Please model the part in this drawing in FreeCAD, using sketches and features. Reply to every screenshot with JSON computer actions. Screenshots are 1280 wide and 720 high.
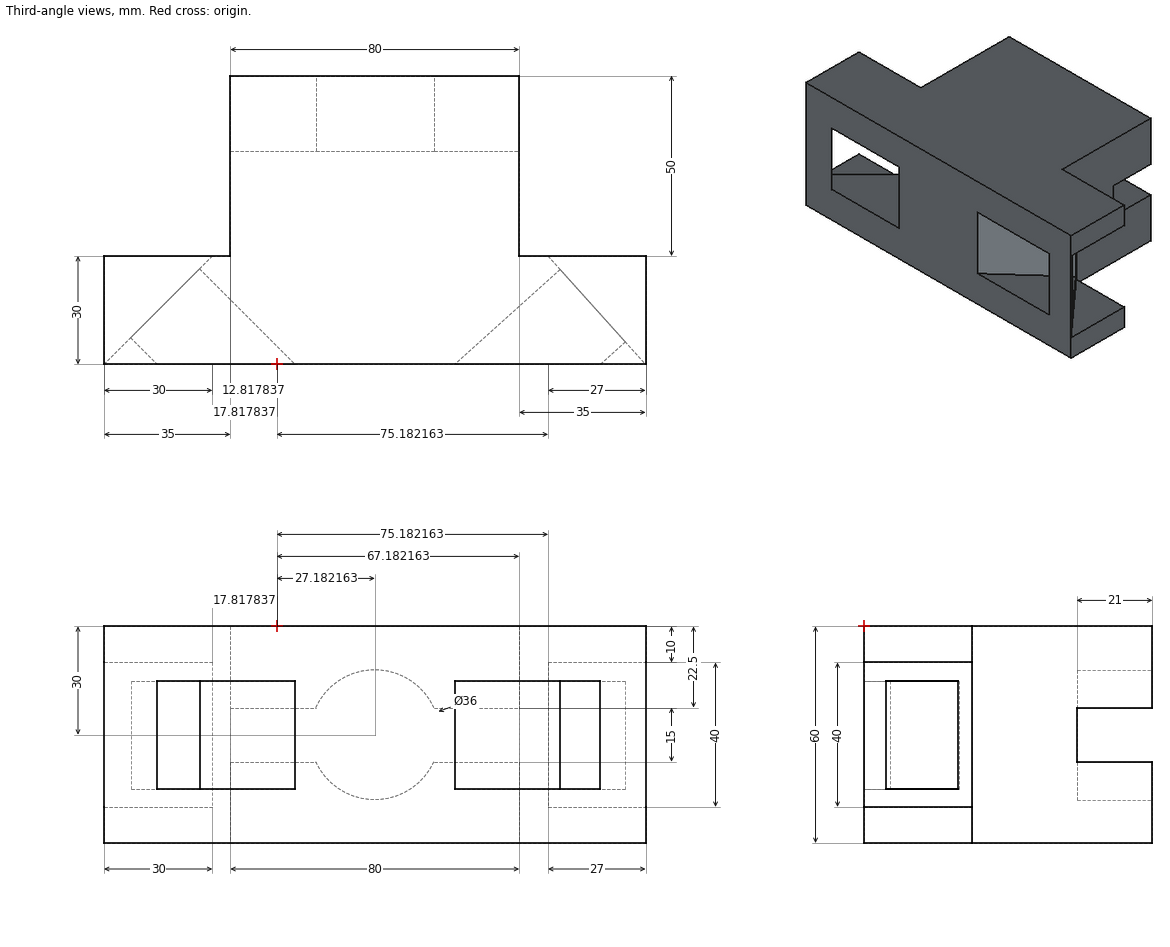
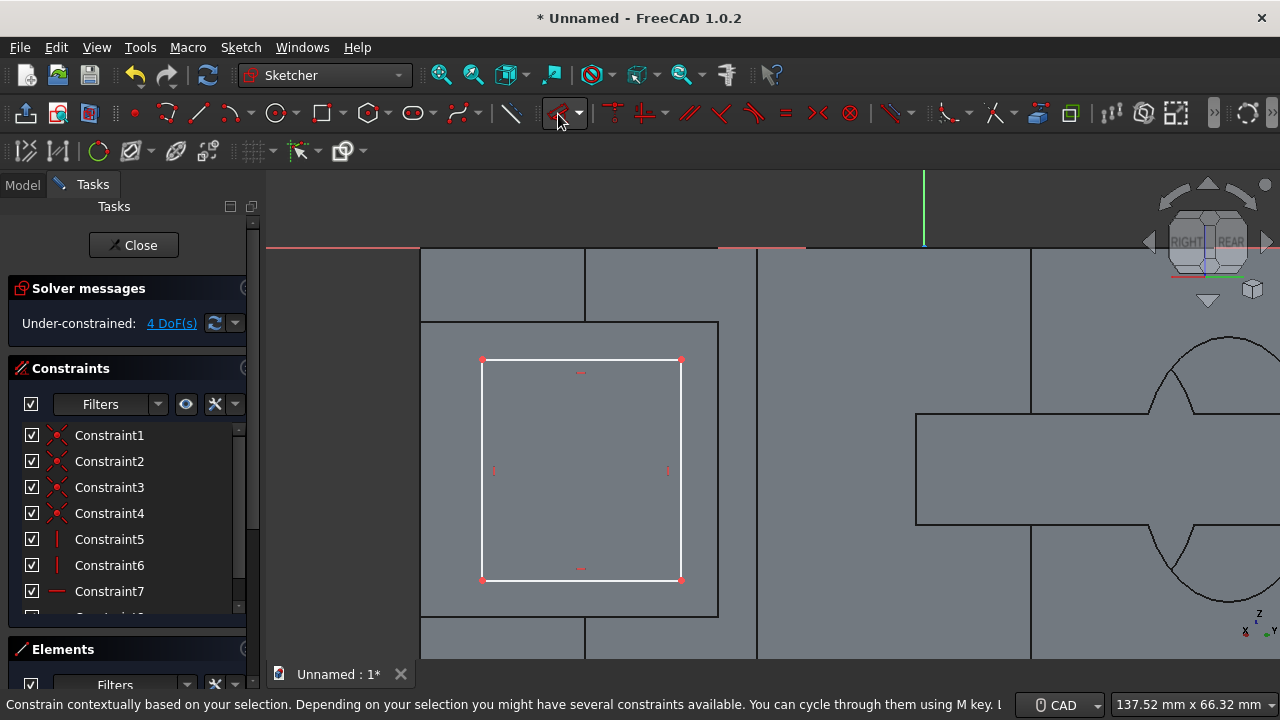
{"action": "left_click", "coordinate": [482, 426]}
{"action": "left_click", "coordinate": [448, 471]}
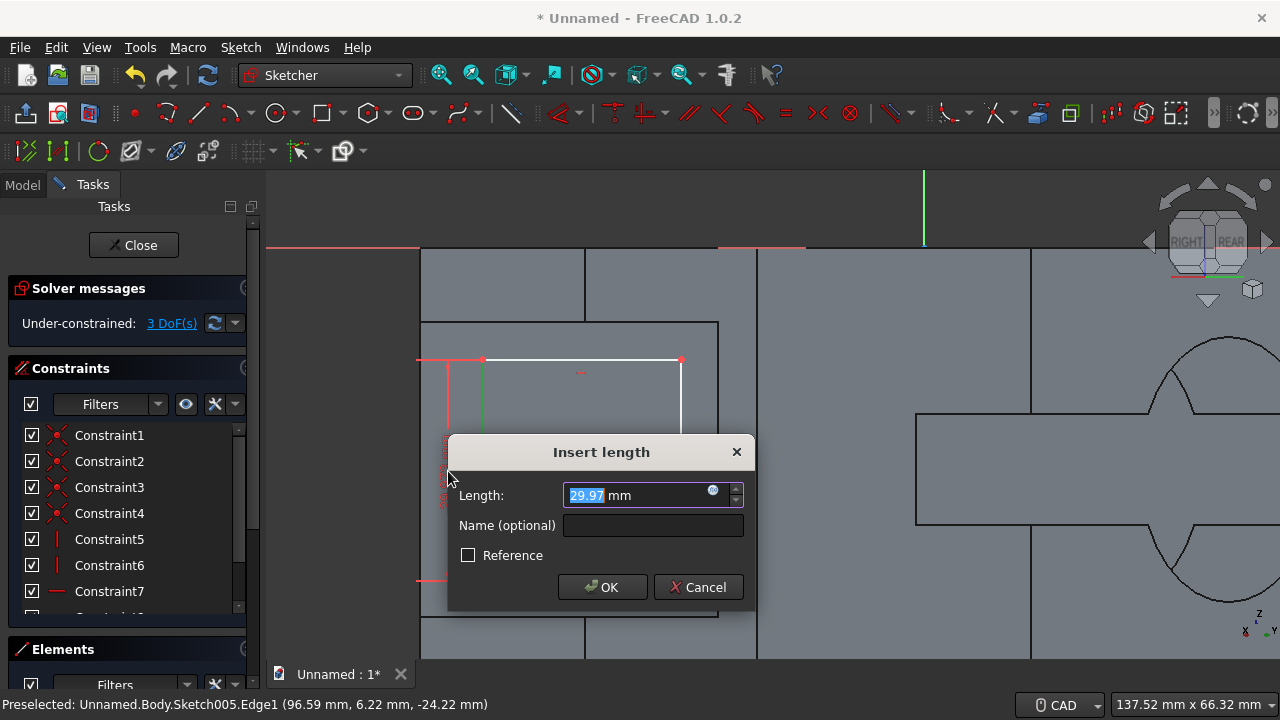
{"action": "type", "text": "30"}
{"action": "key", "text": "Return"}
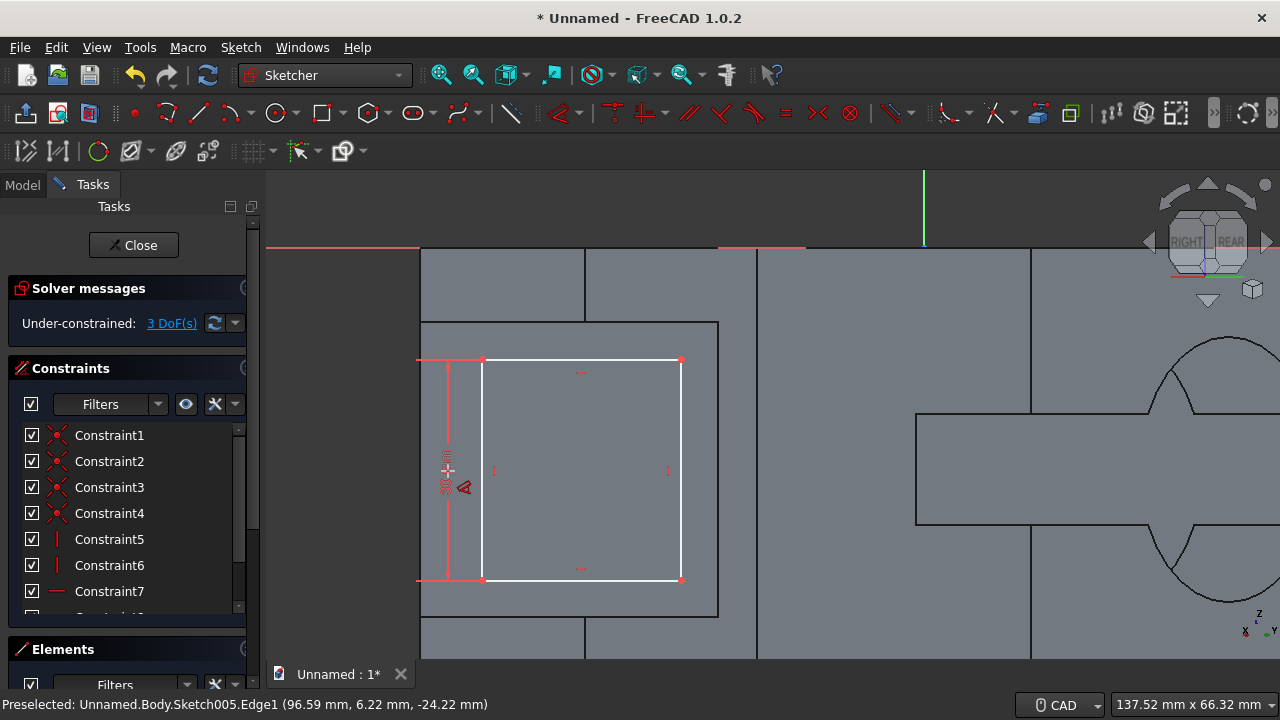
{"action": "left_click", "coordinate": [542, 581]}
{"action": "left_click", "coordinate": [581, 615]}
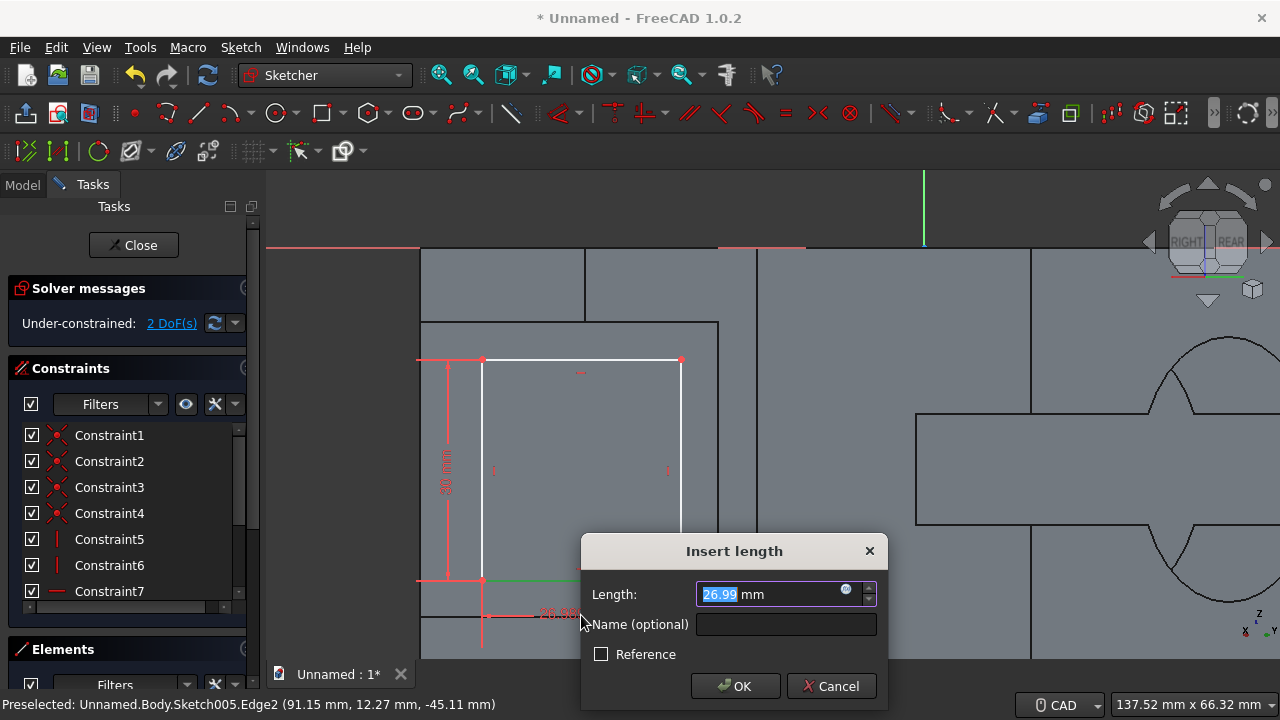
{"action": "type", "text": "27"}
{"action": "key", "text": "Return"}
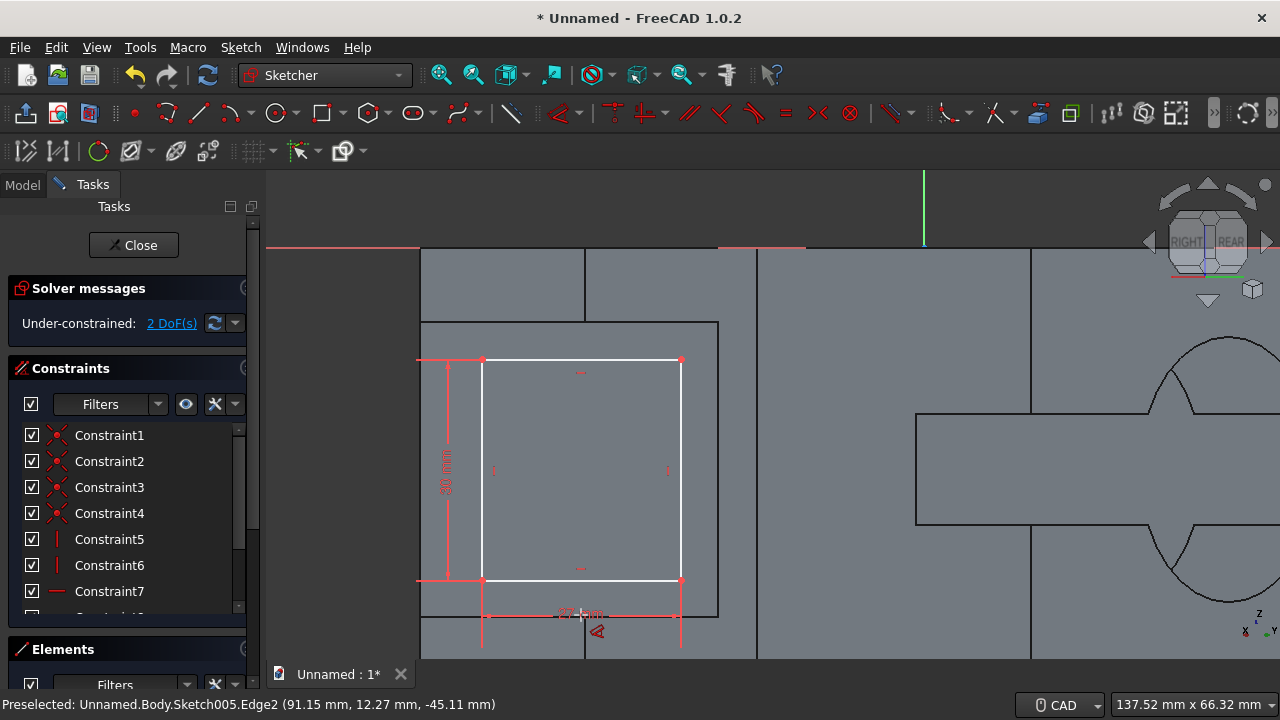
{"action": "left_click", "coordinate": [482, 360]}
{"action": "left_click", "coordinate": [958, 304]}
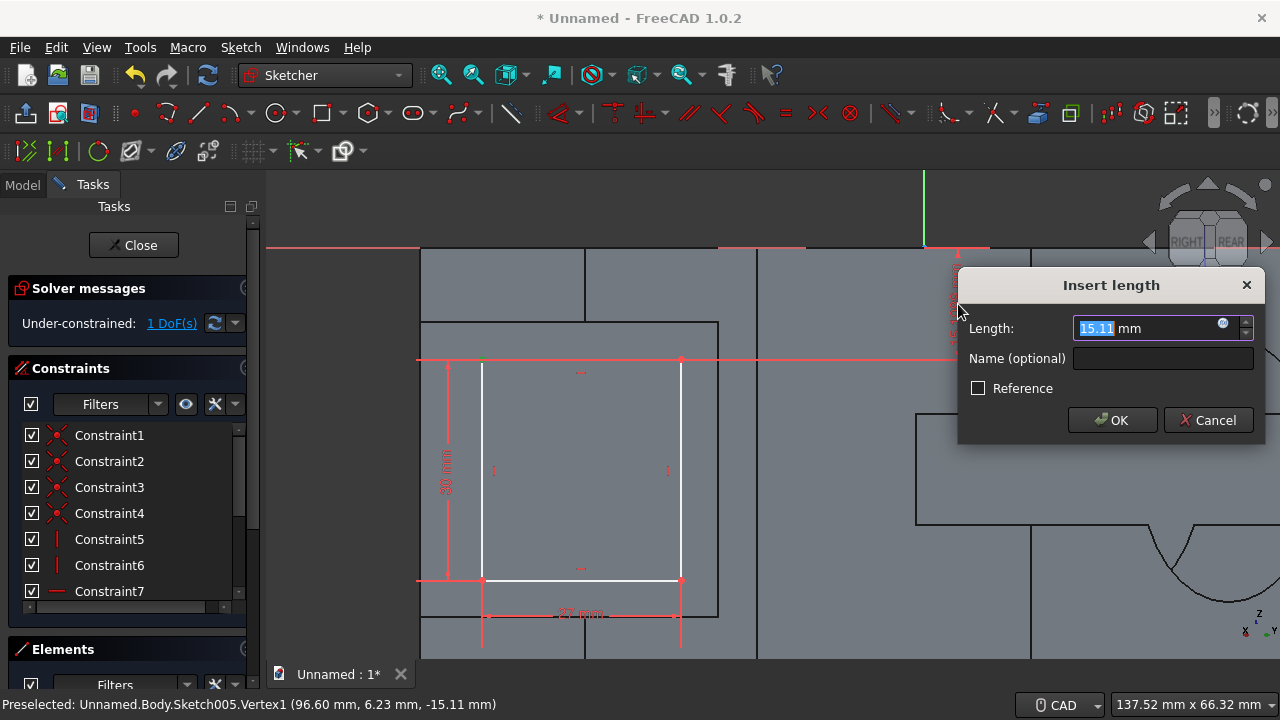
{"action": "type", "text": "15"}
{"action": "key", "text": "Return"}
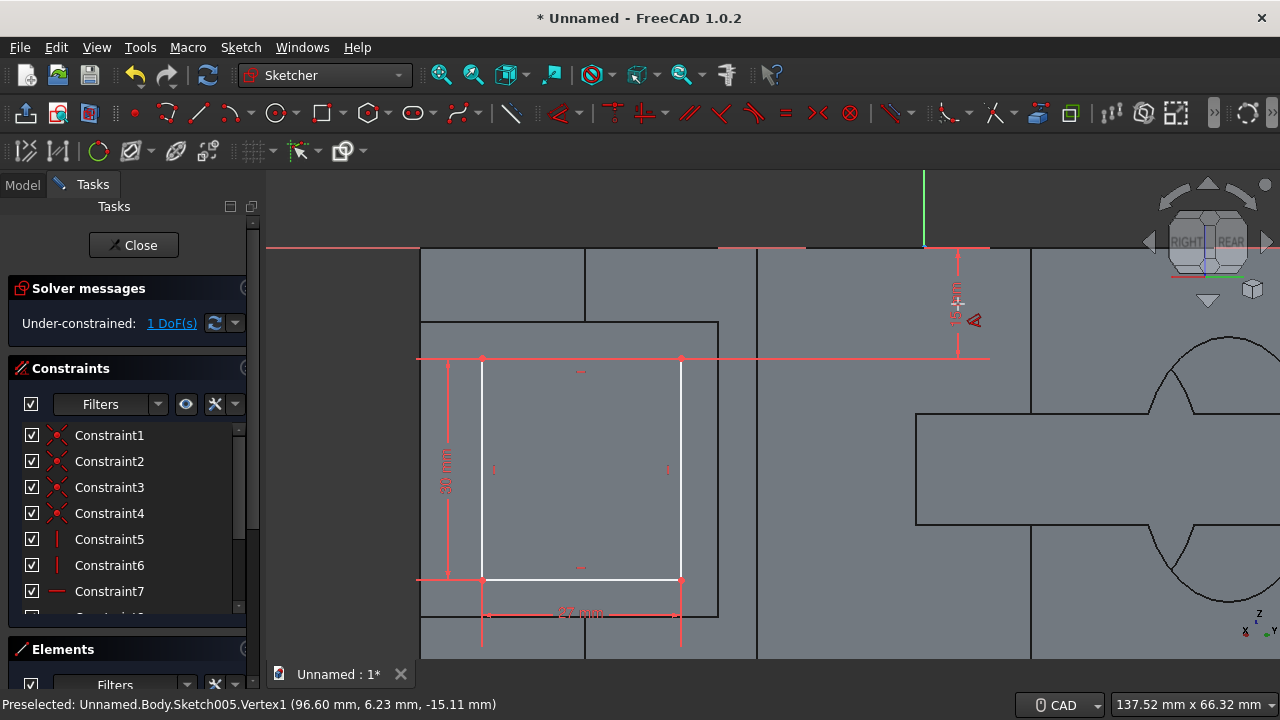
{"action": "left_click", "coordinate": [482, 359]}
{"action": "left_click", "coordinate": [703, 214]}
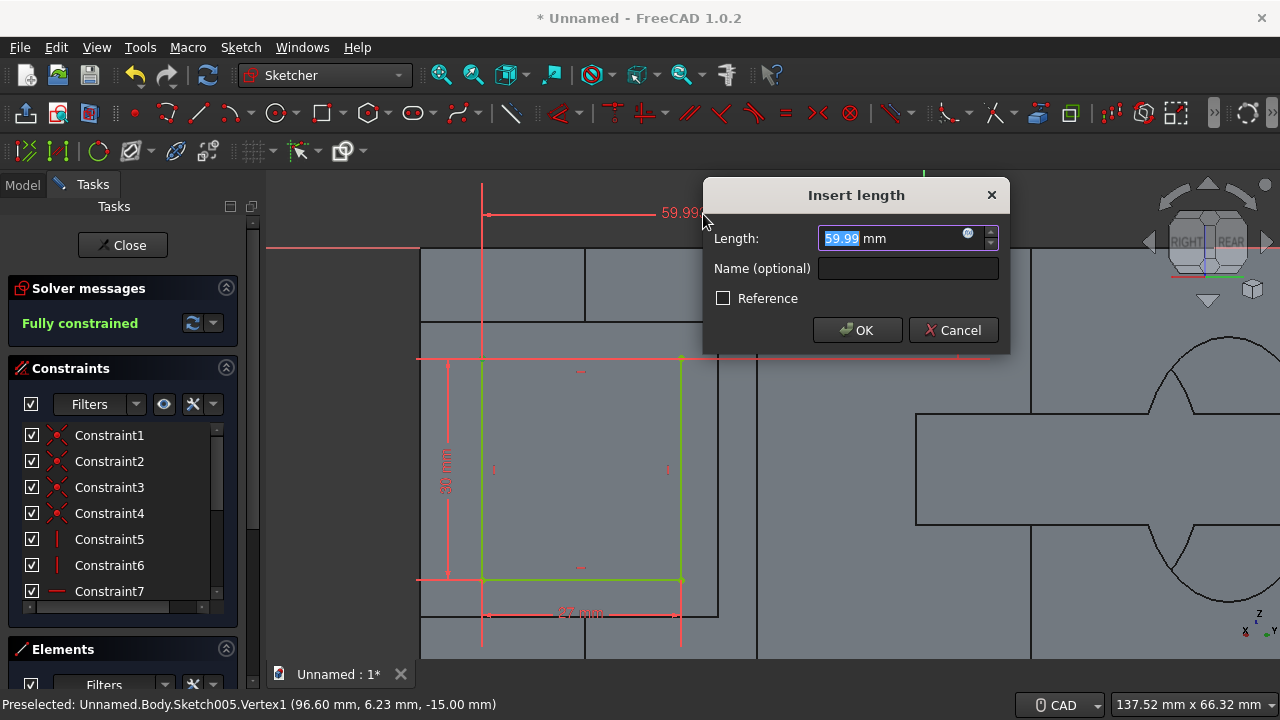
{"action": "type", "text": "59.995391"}
{"action": "key", "text": "Return"}
{"action": "key", "text": "Escape"}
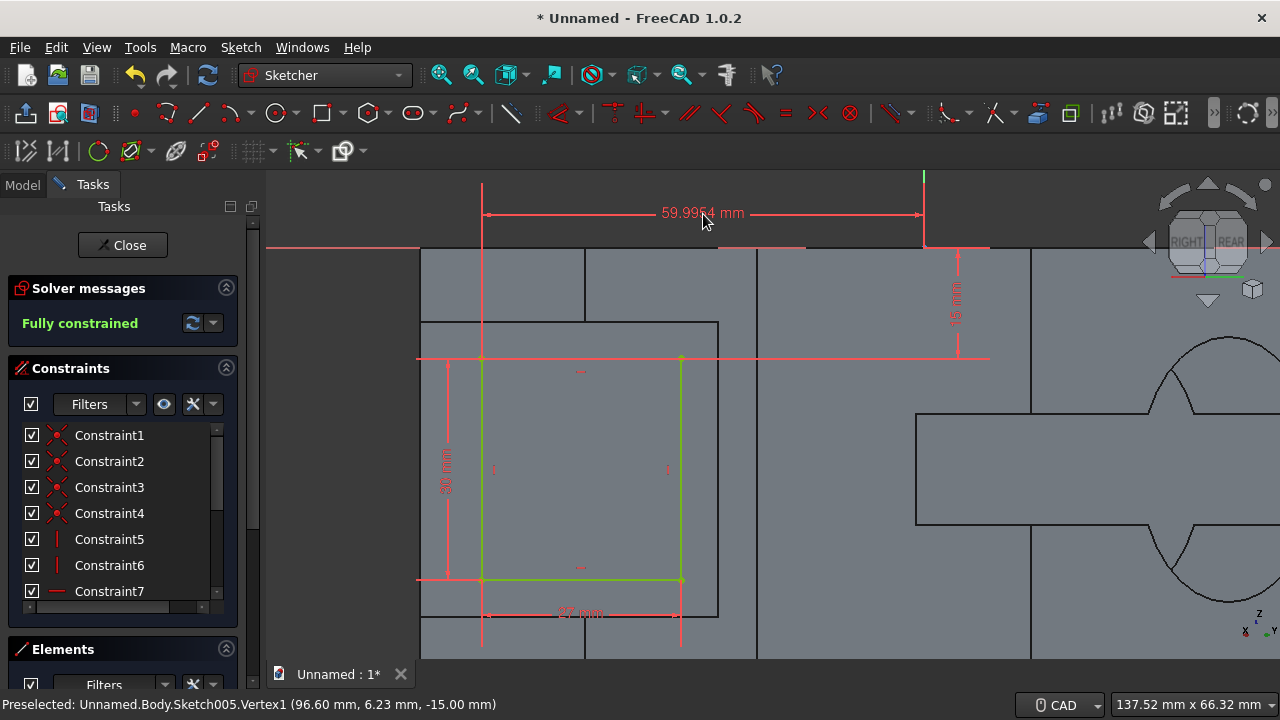
{"action": "left_click", "coordinate": [123, 245]}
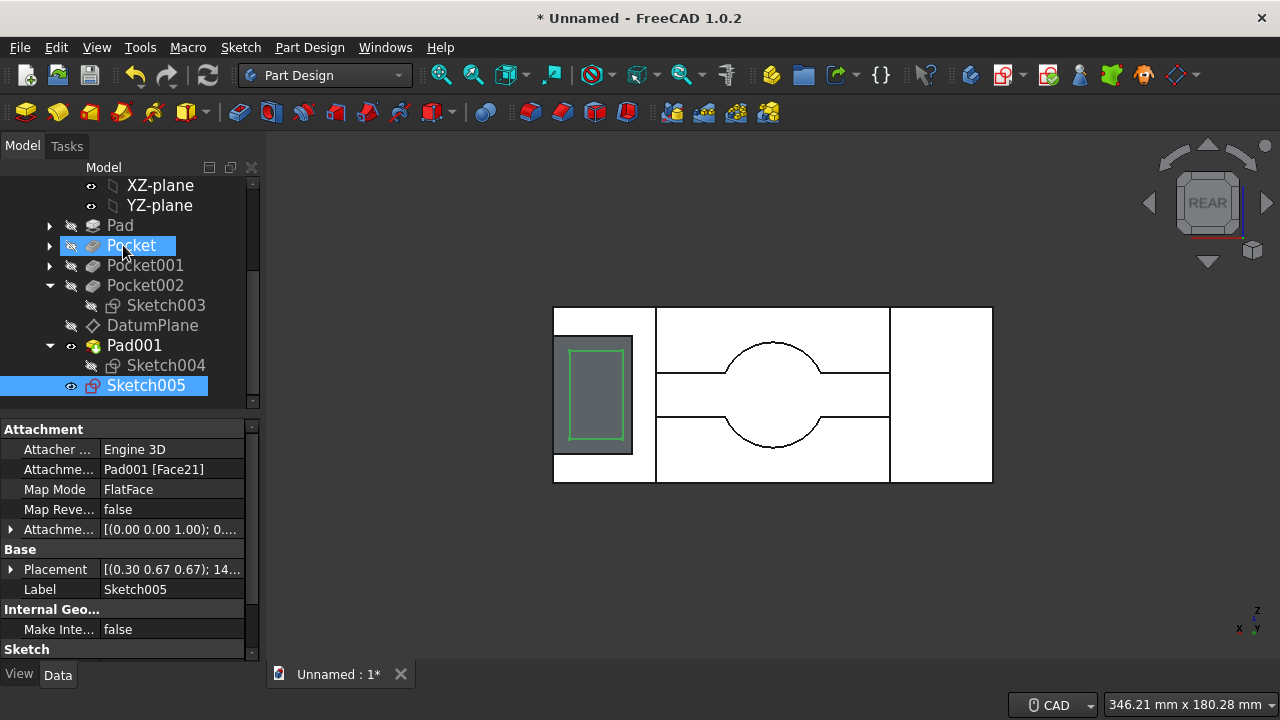
{"action": "left_click", "coordinate": [240, 112]}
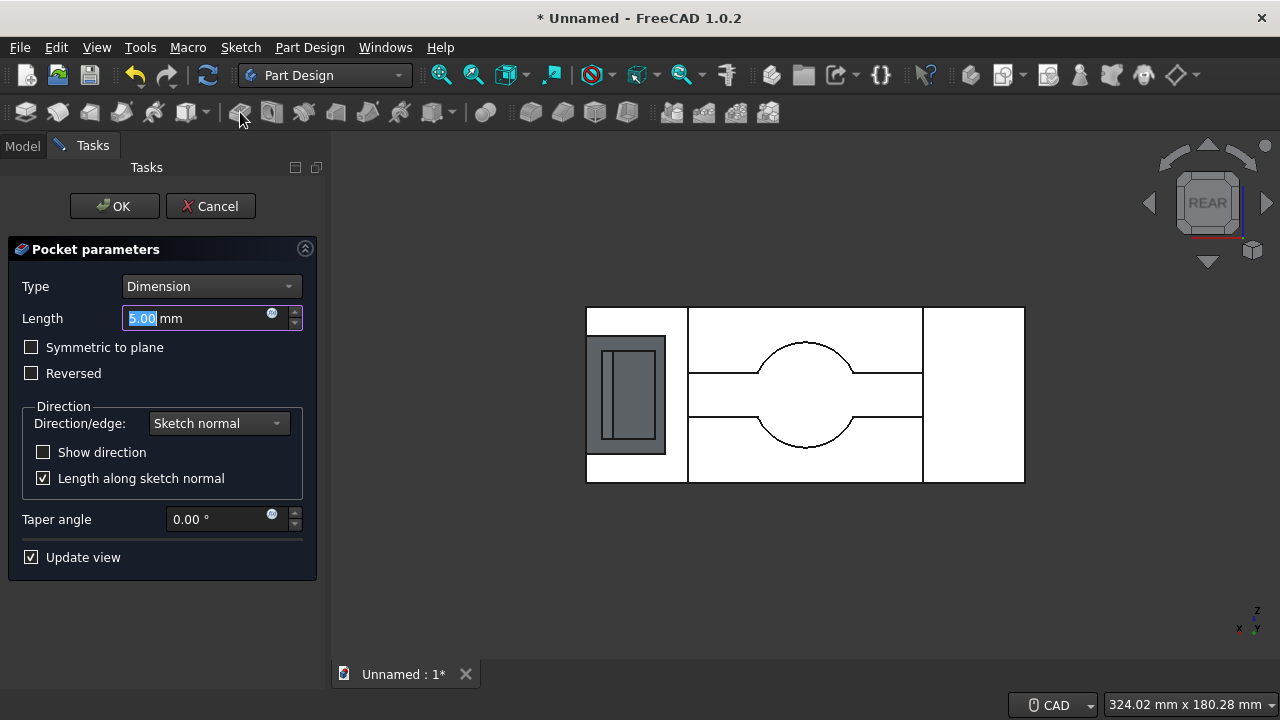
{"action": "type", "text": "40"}
{"action": "key", "text": "Tab"}